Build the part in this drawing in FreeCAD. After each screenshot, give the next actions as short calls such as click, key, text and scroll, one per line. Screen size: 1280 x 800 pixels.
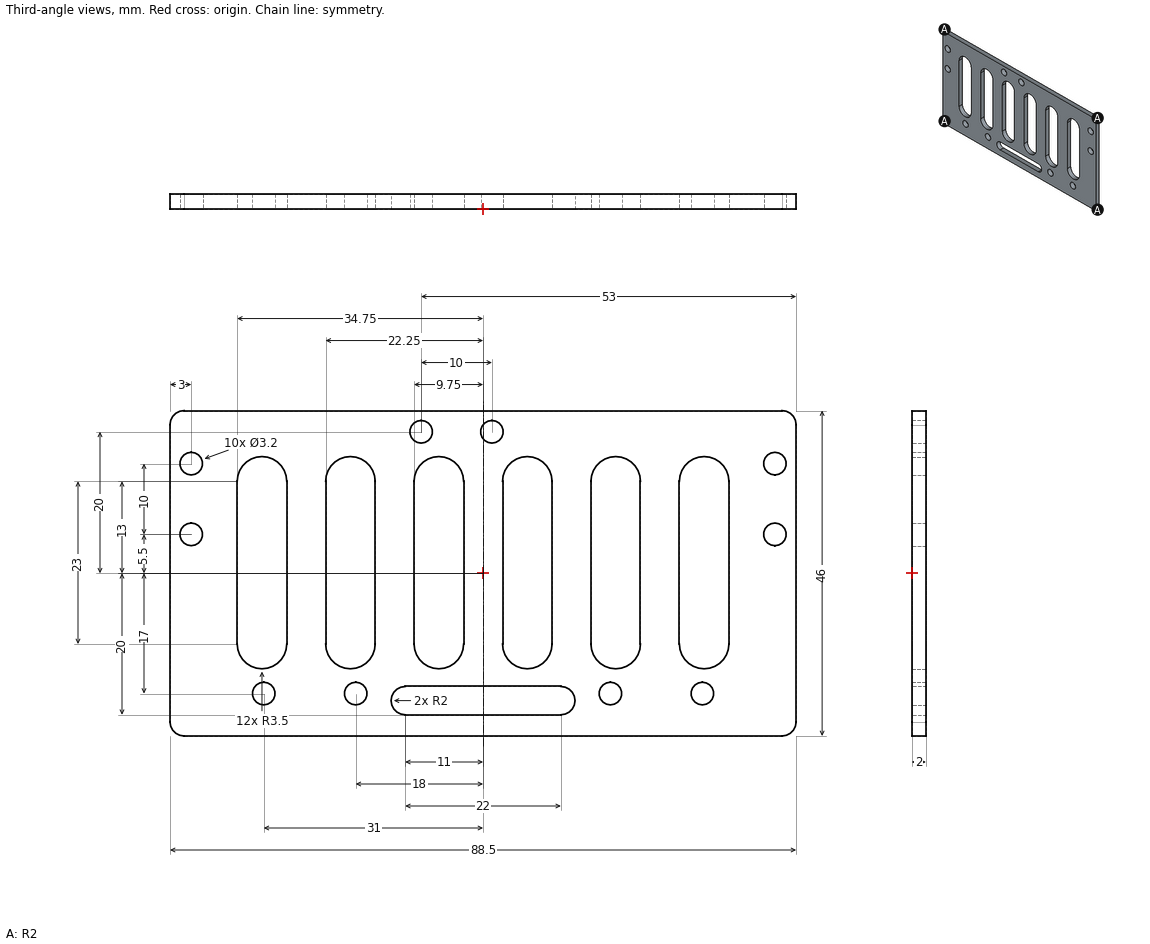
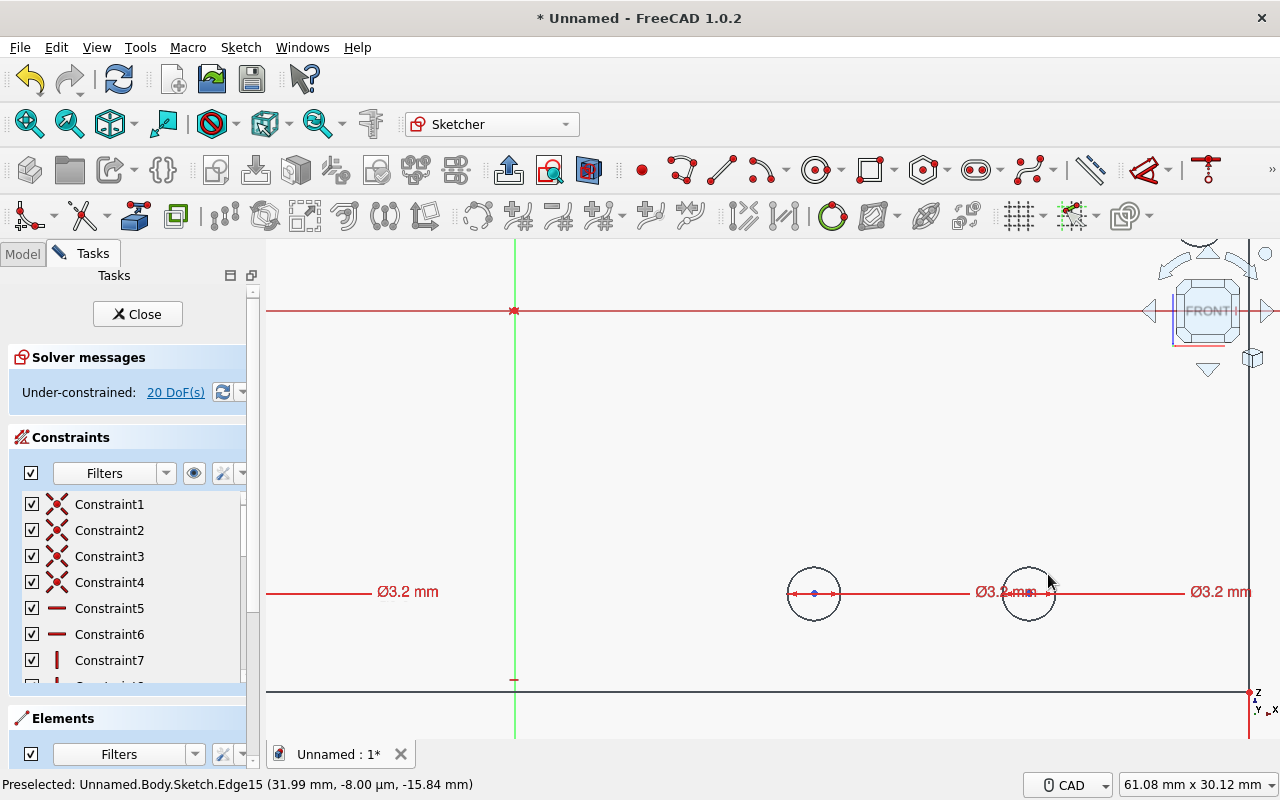
scroll(815, 593, down, 5)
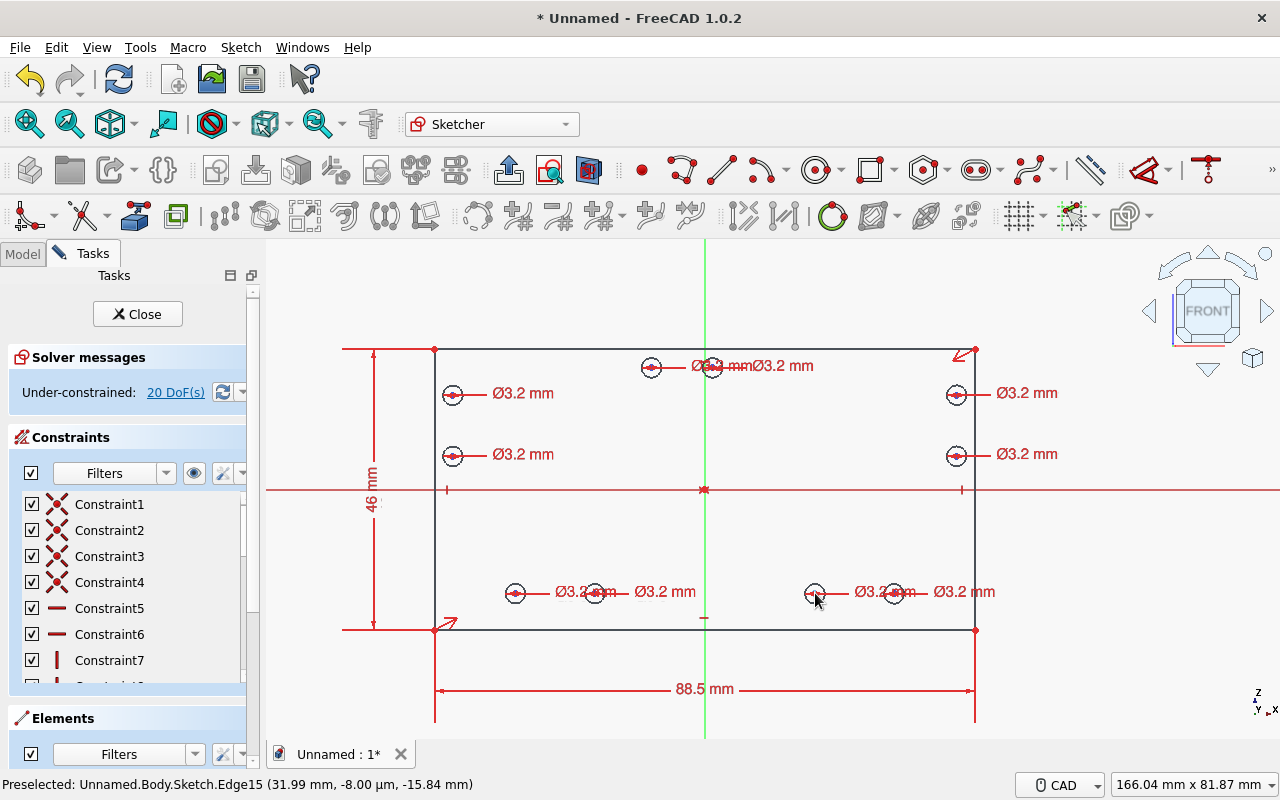
click(453, 395)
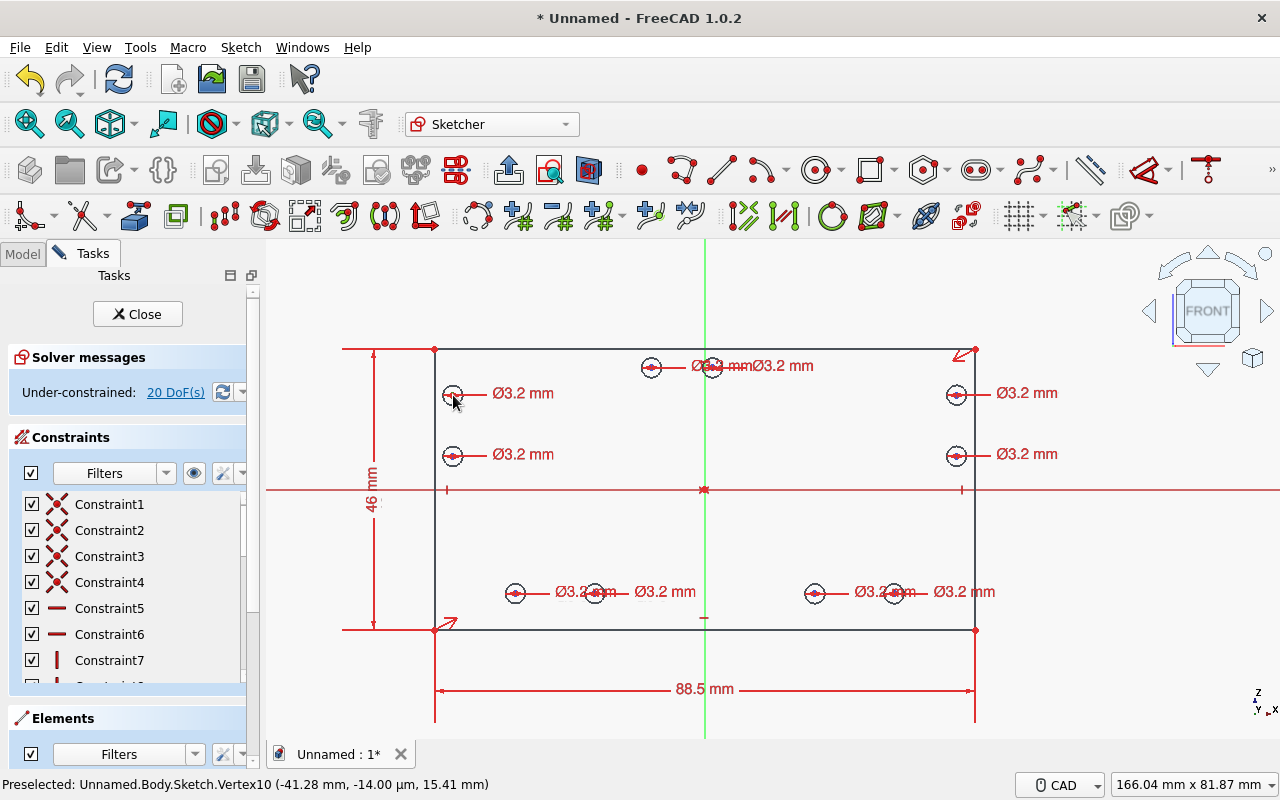
click(957, 395)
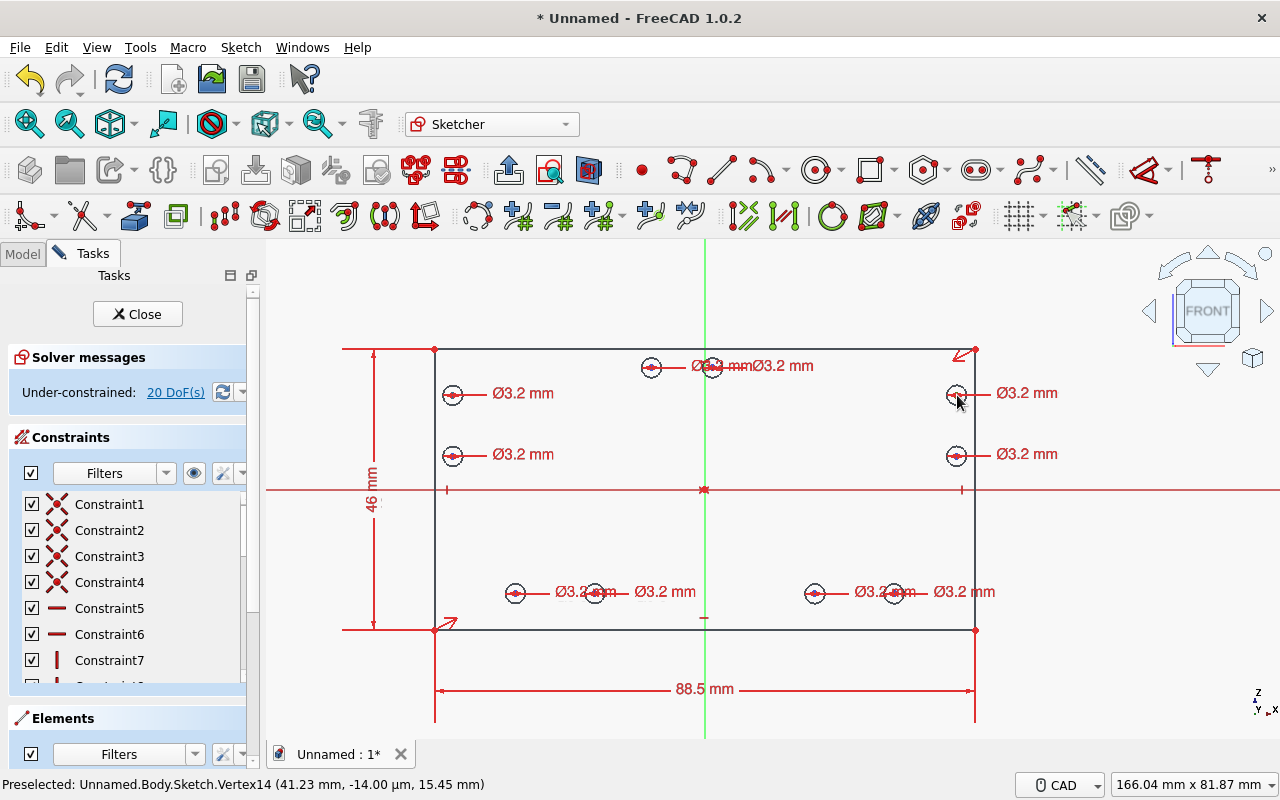
click(705, 679)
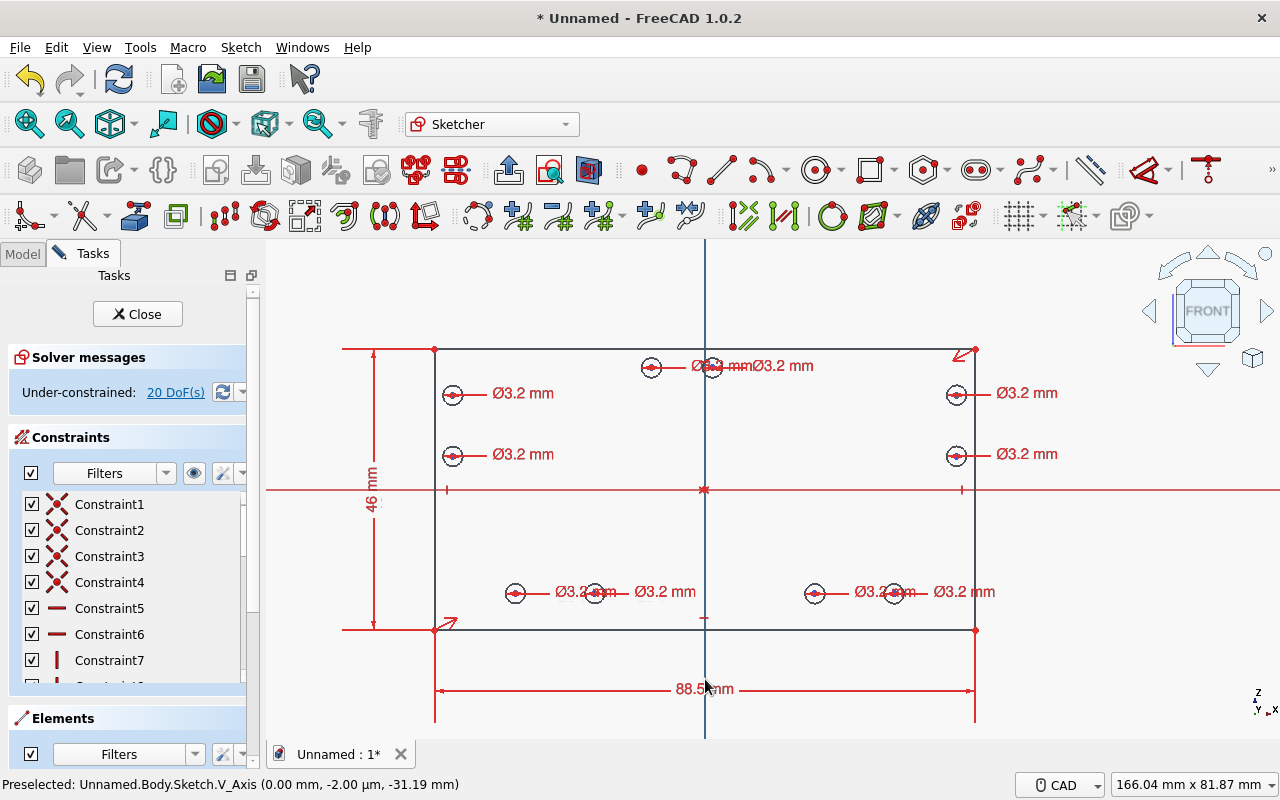
key(s)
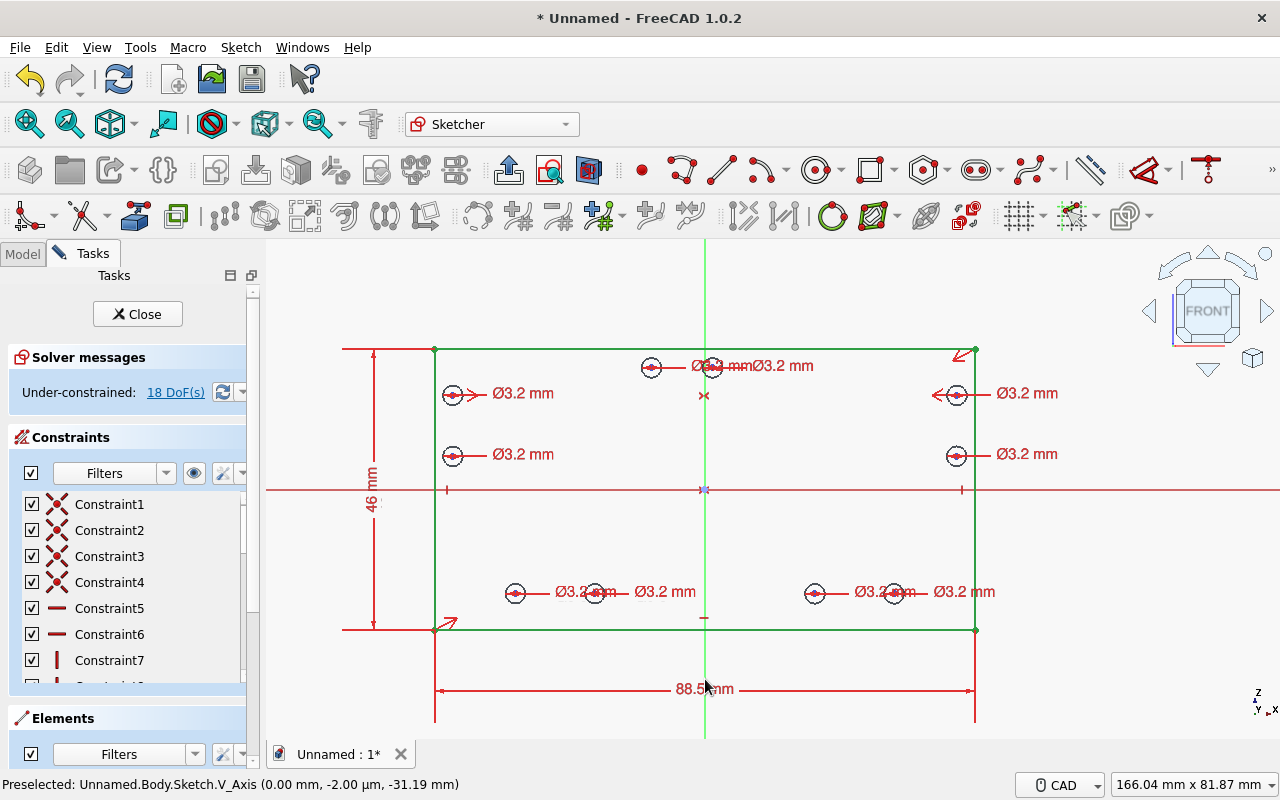
click(453, 456)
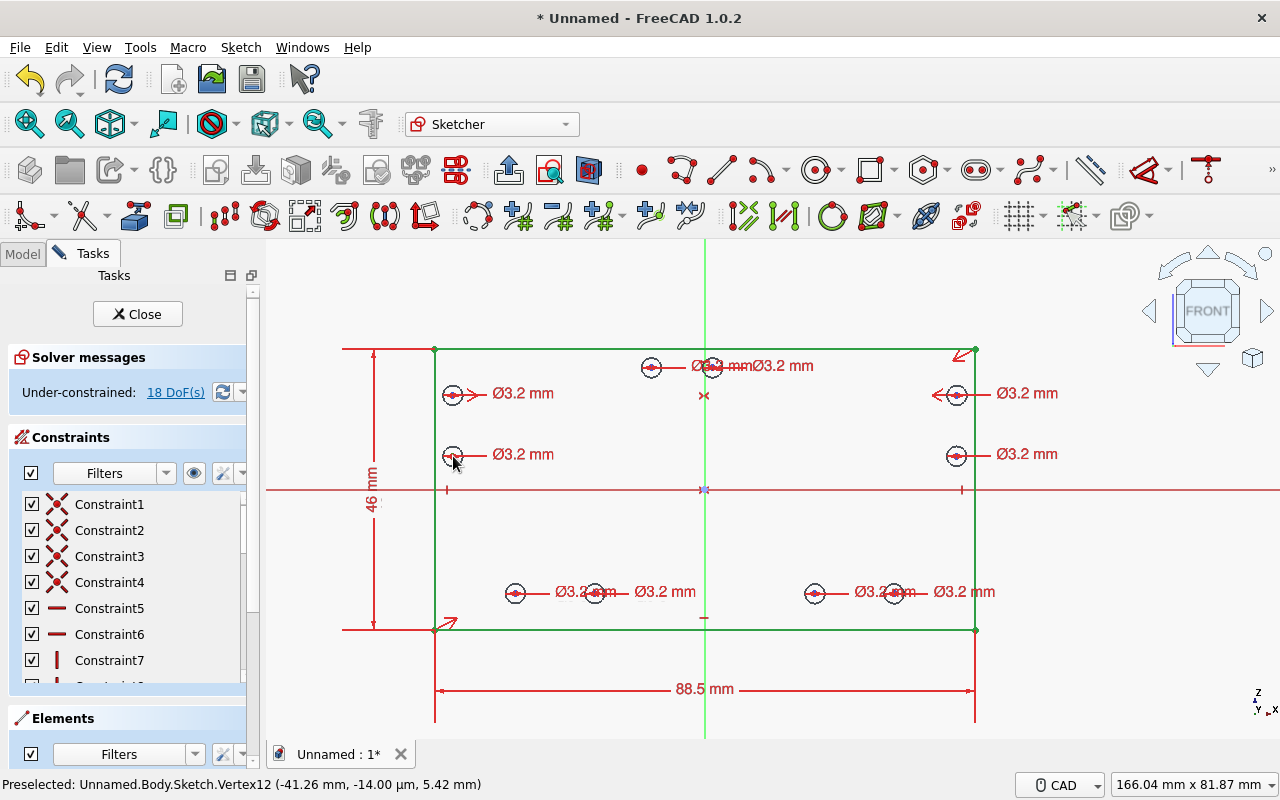
click(957, 456)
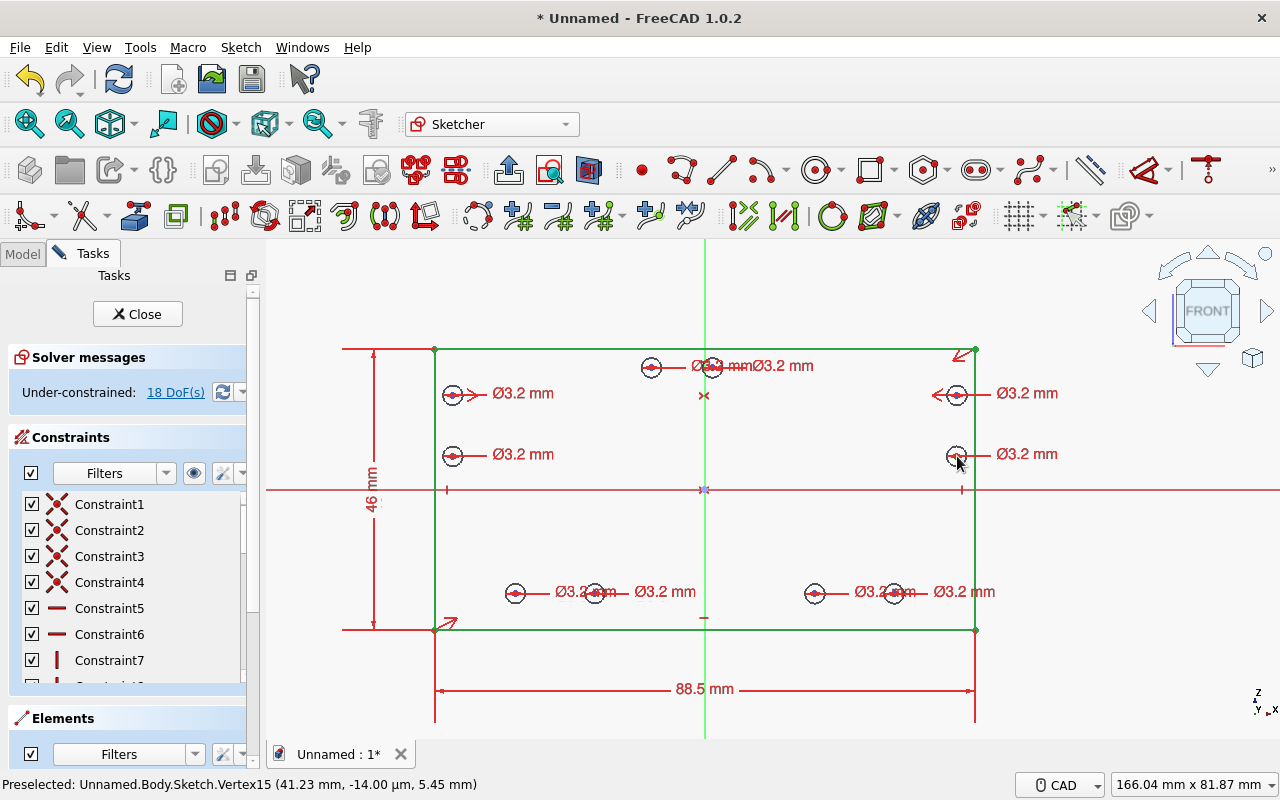
click(705, 679)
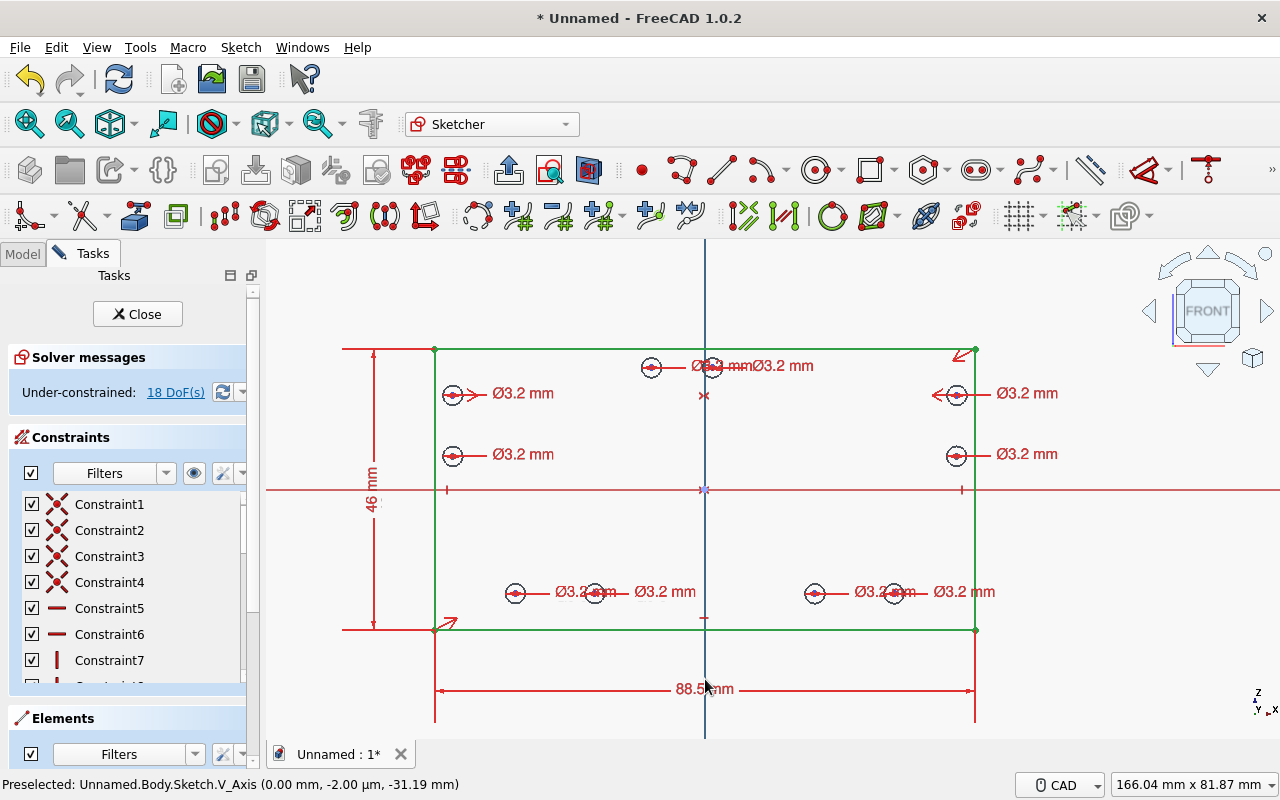
key(s)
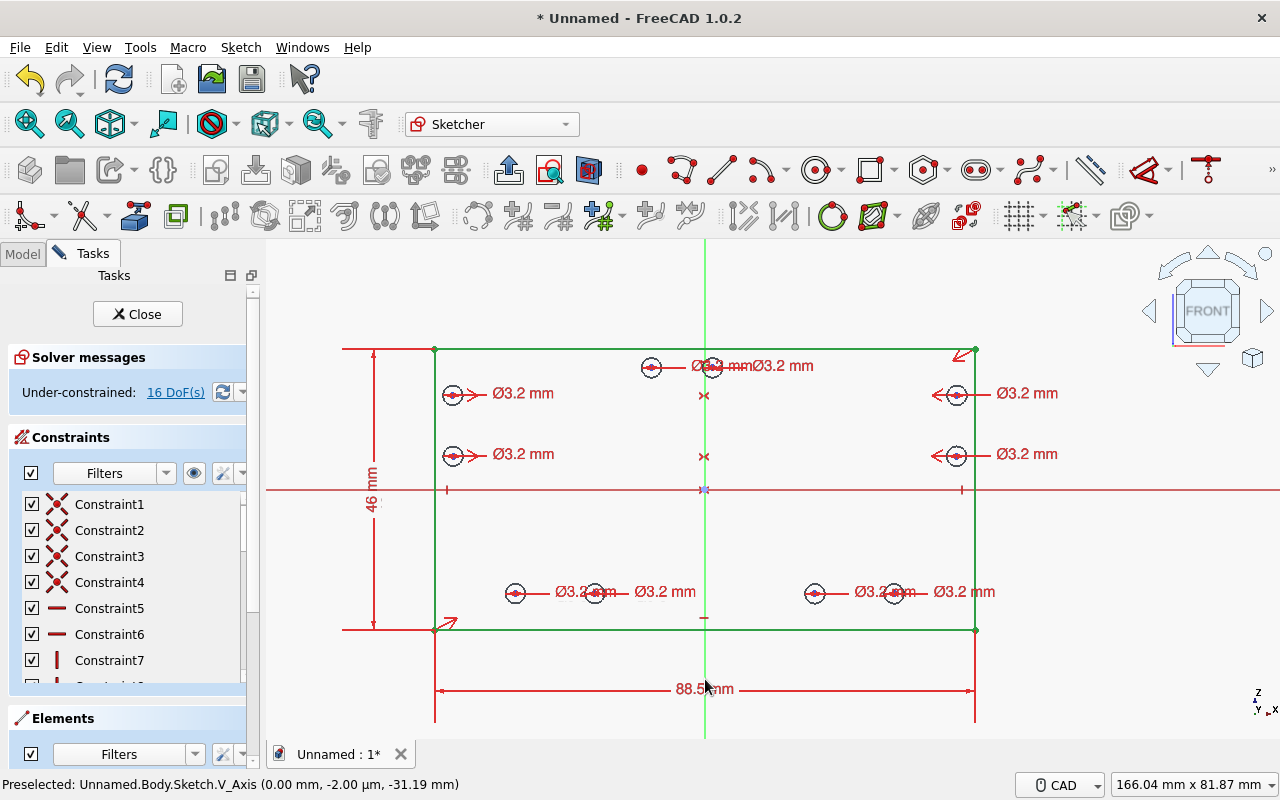
click(595, 594)